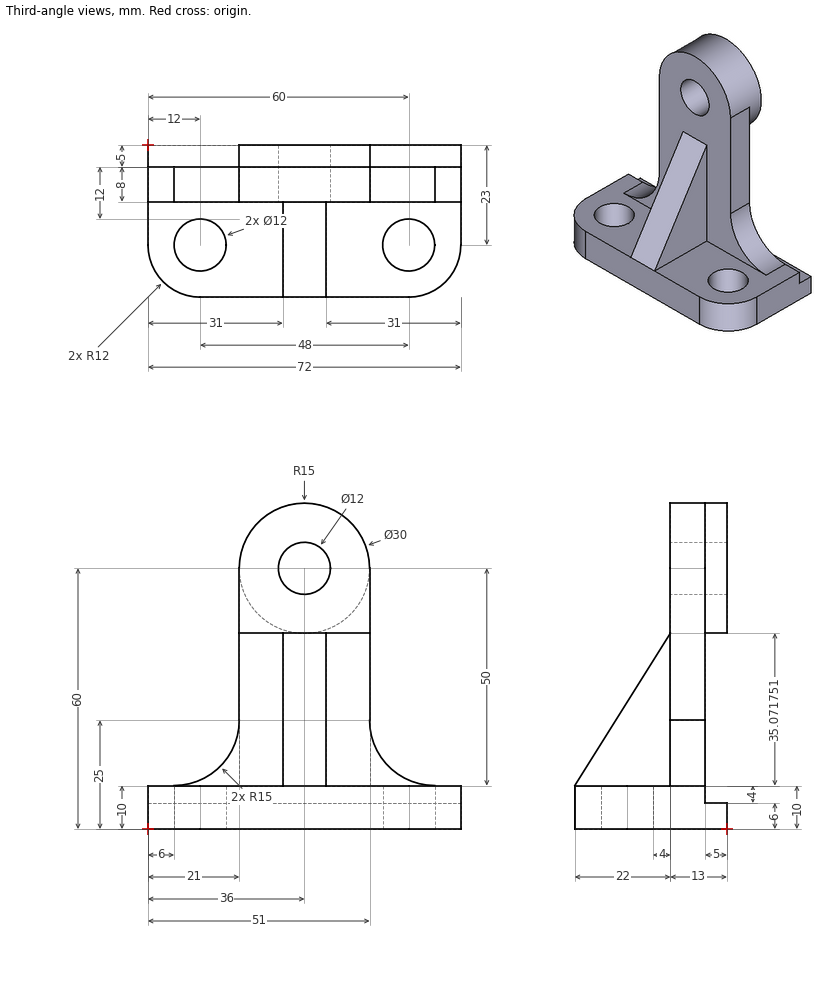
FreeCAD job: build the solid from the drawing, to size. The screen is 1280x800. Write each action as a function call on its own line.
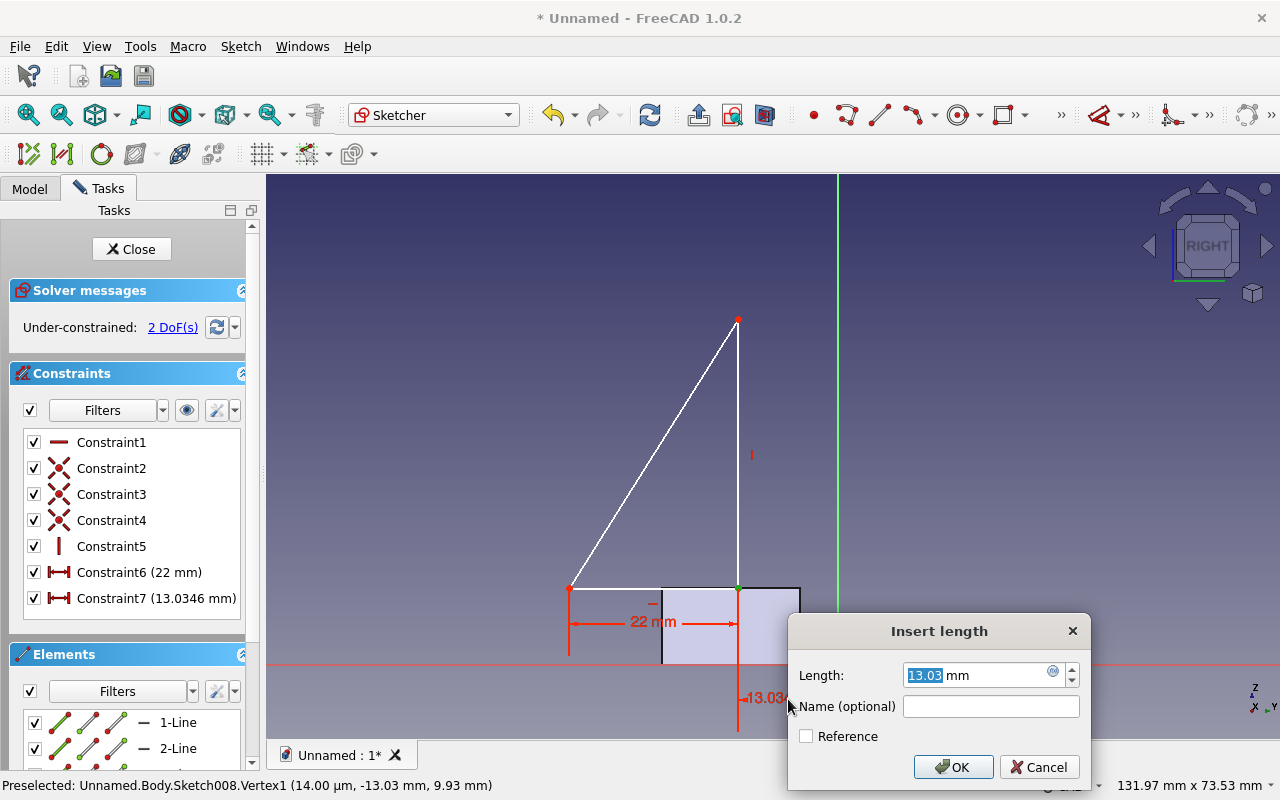
text(13)
key(Return)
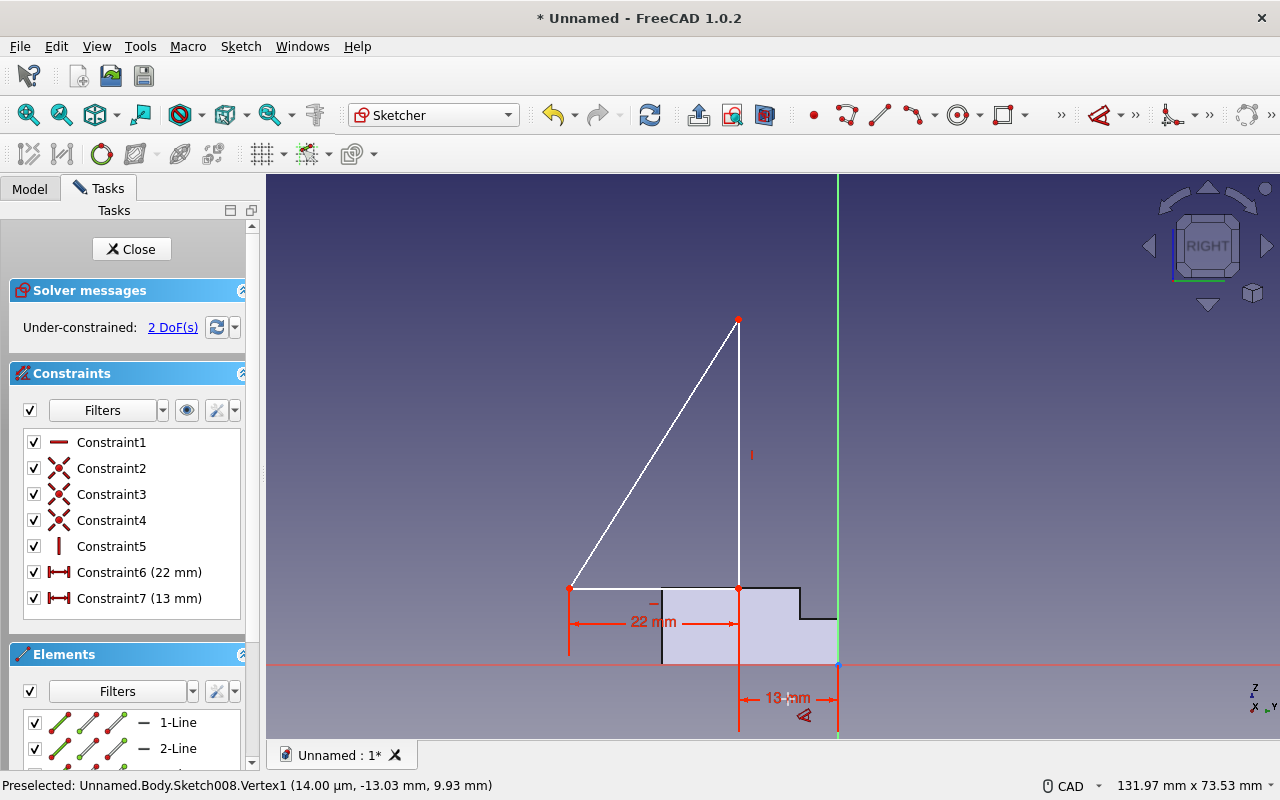
click(739, 589)
click(872, 627)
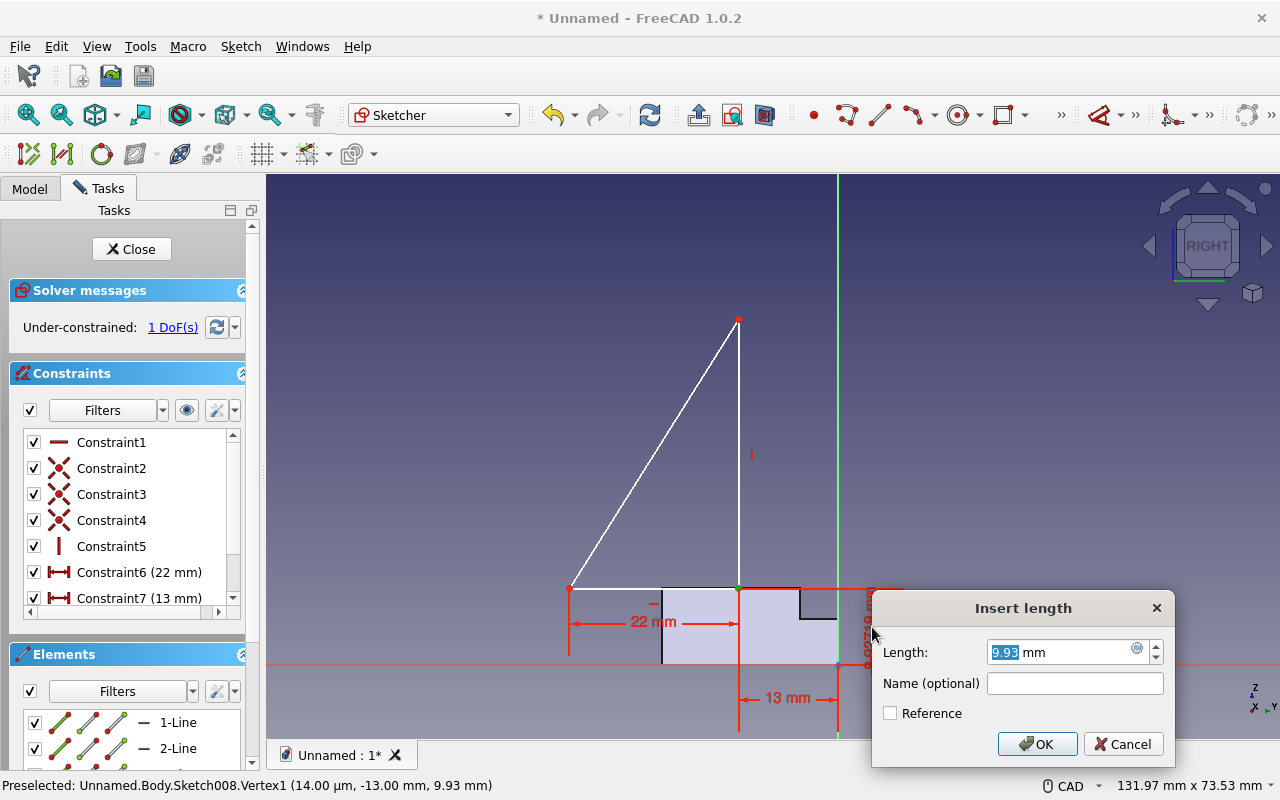
text(10)
key(Return)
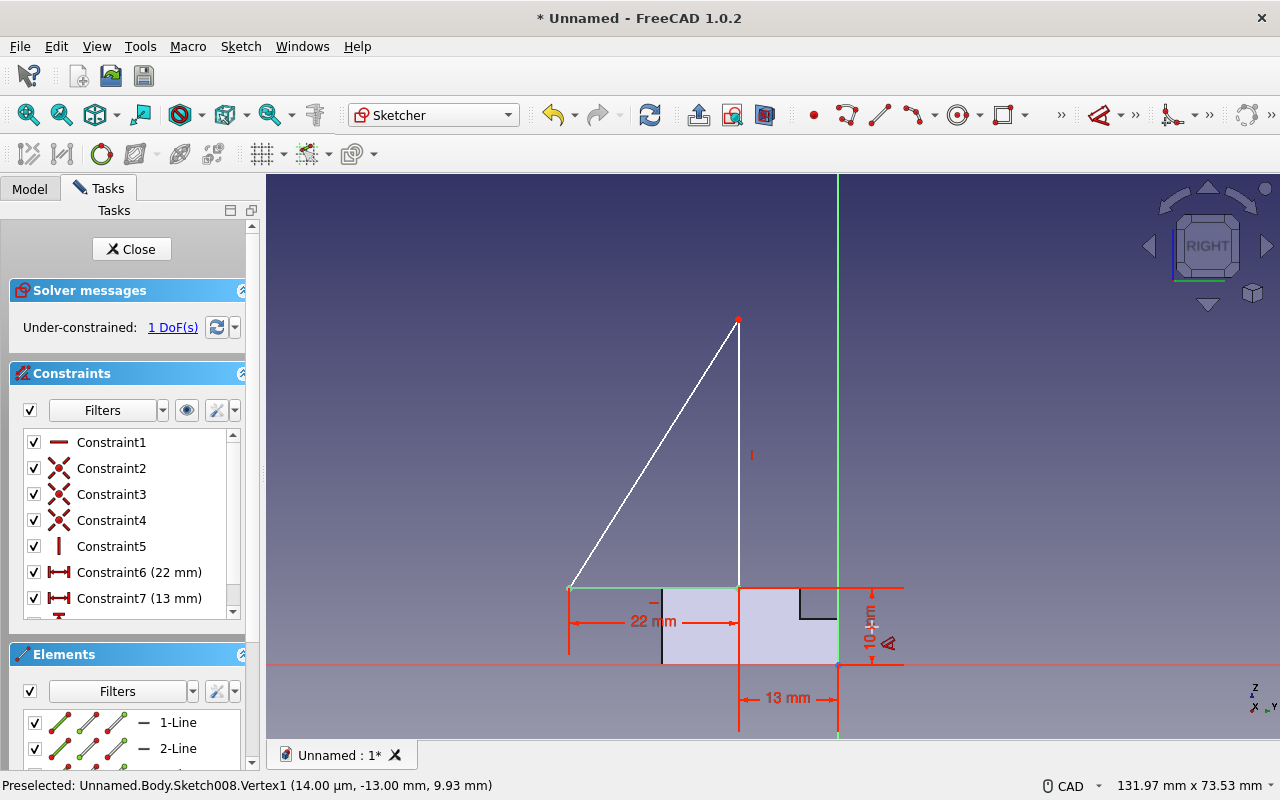
click(739, 401)
click(773, 454)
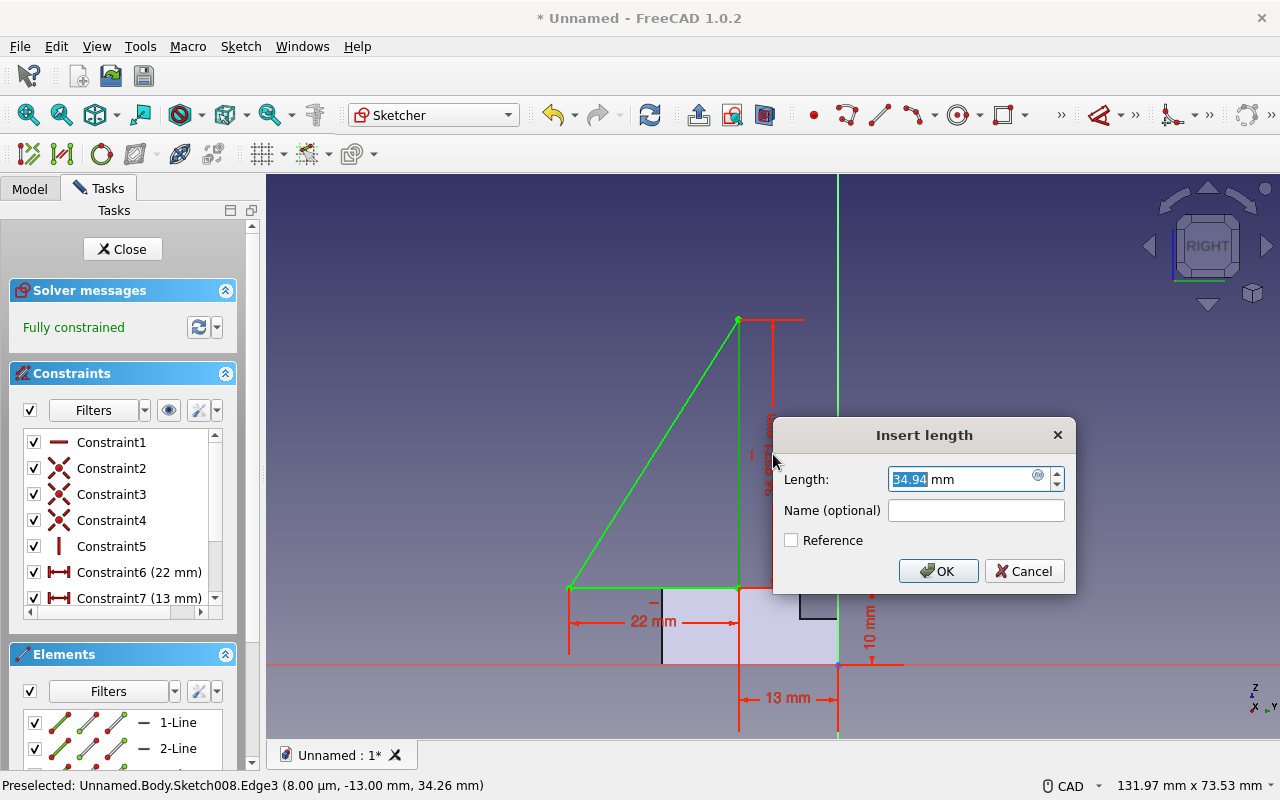
text(35.071751)
key(Return)
key(Escape)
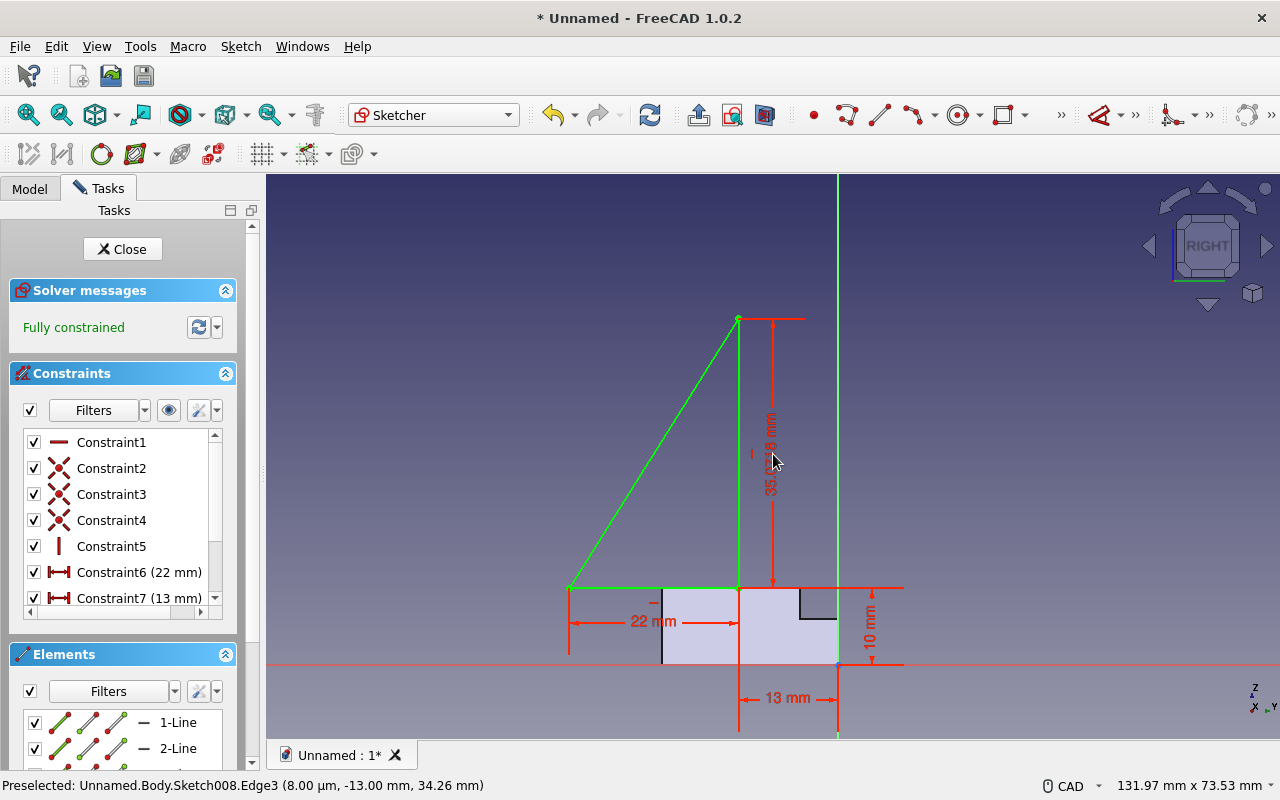
click(123, 249)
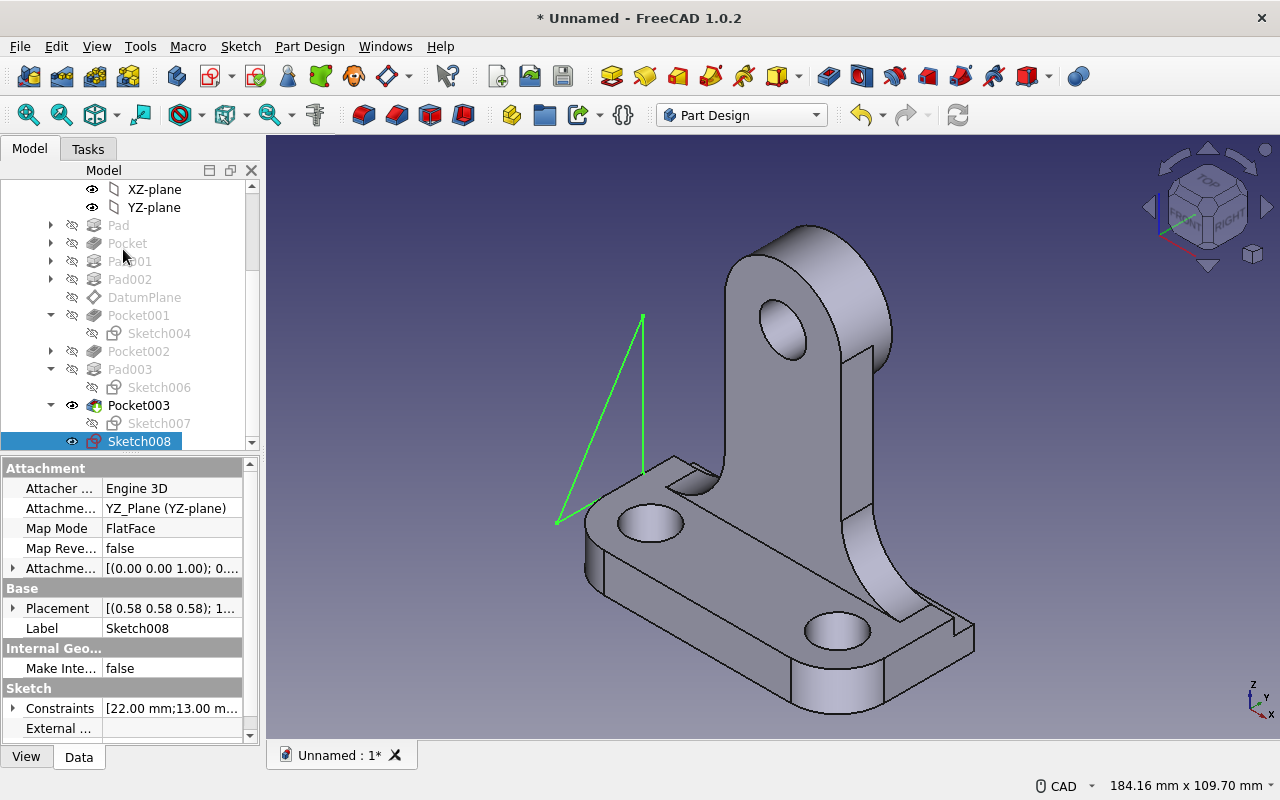
click(612, 76)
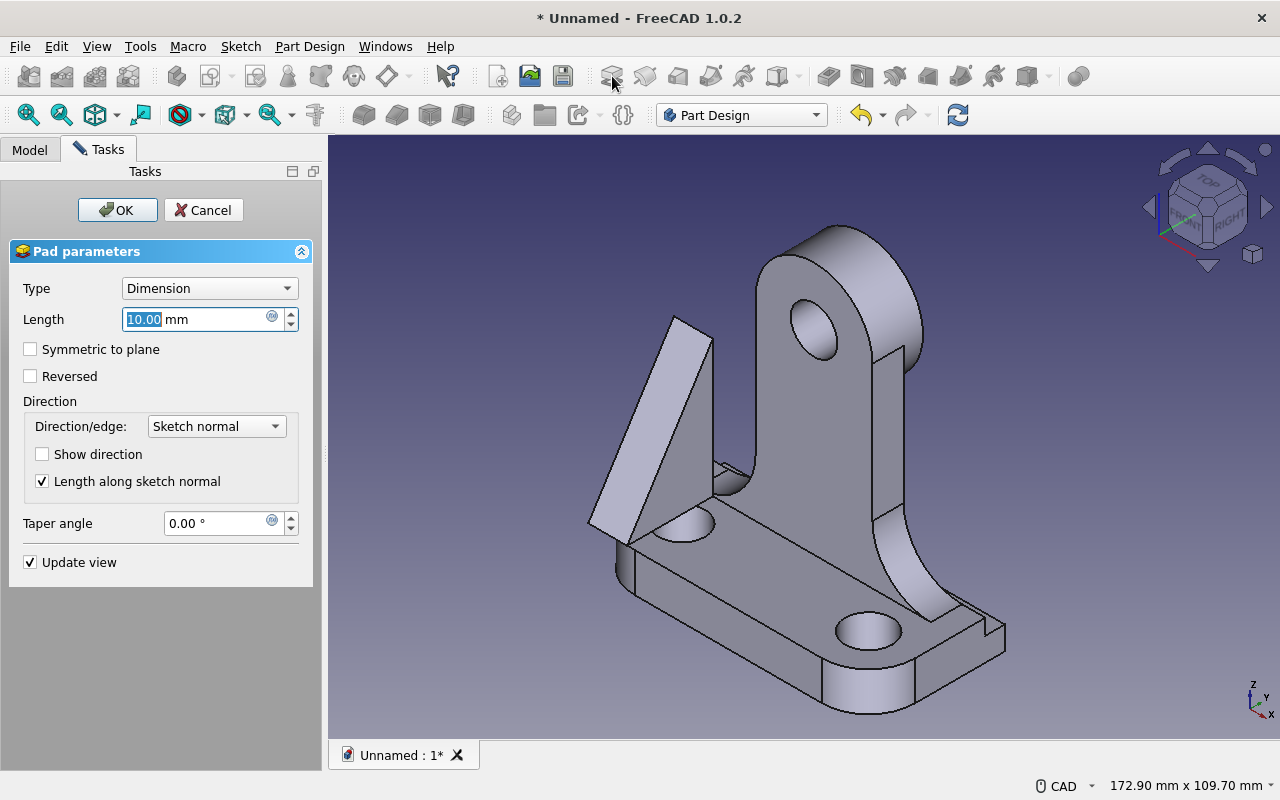
text(72)
key(Tab)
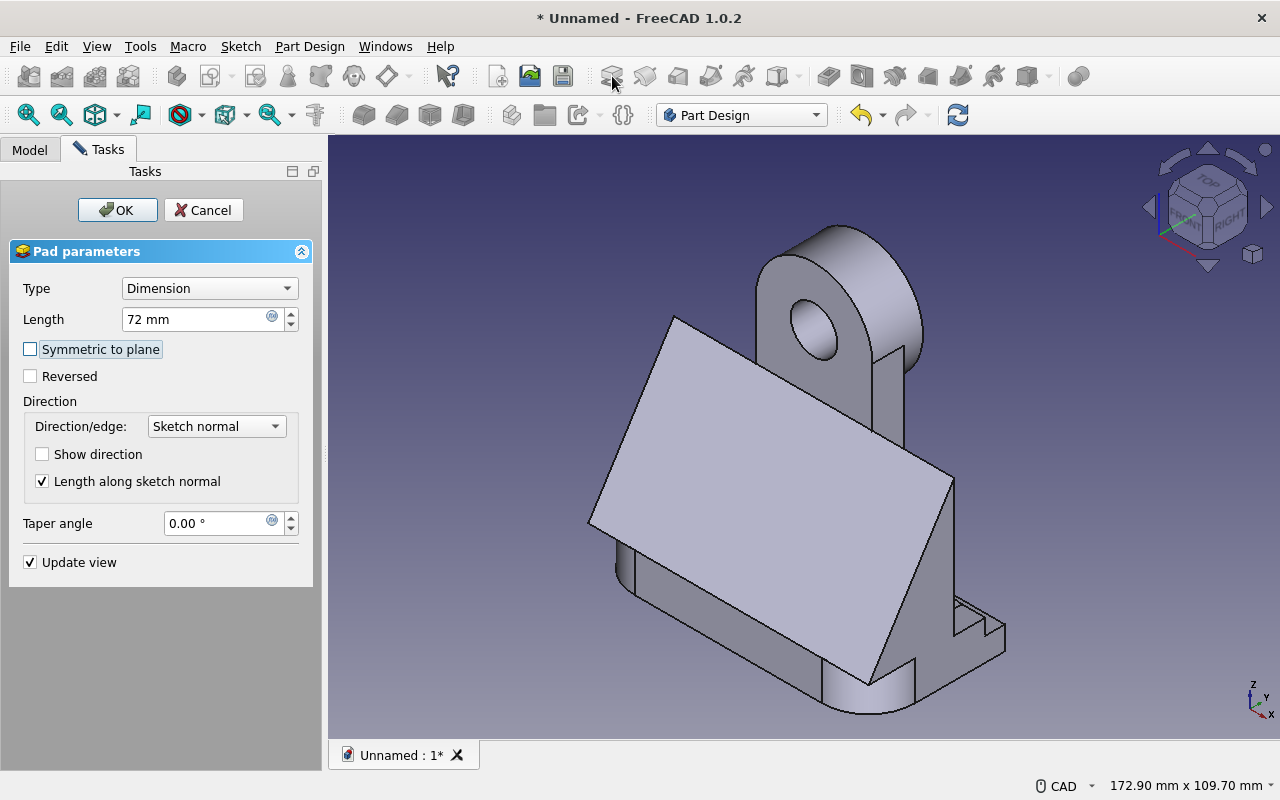
click(118, 210)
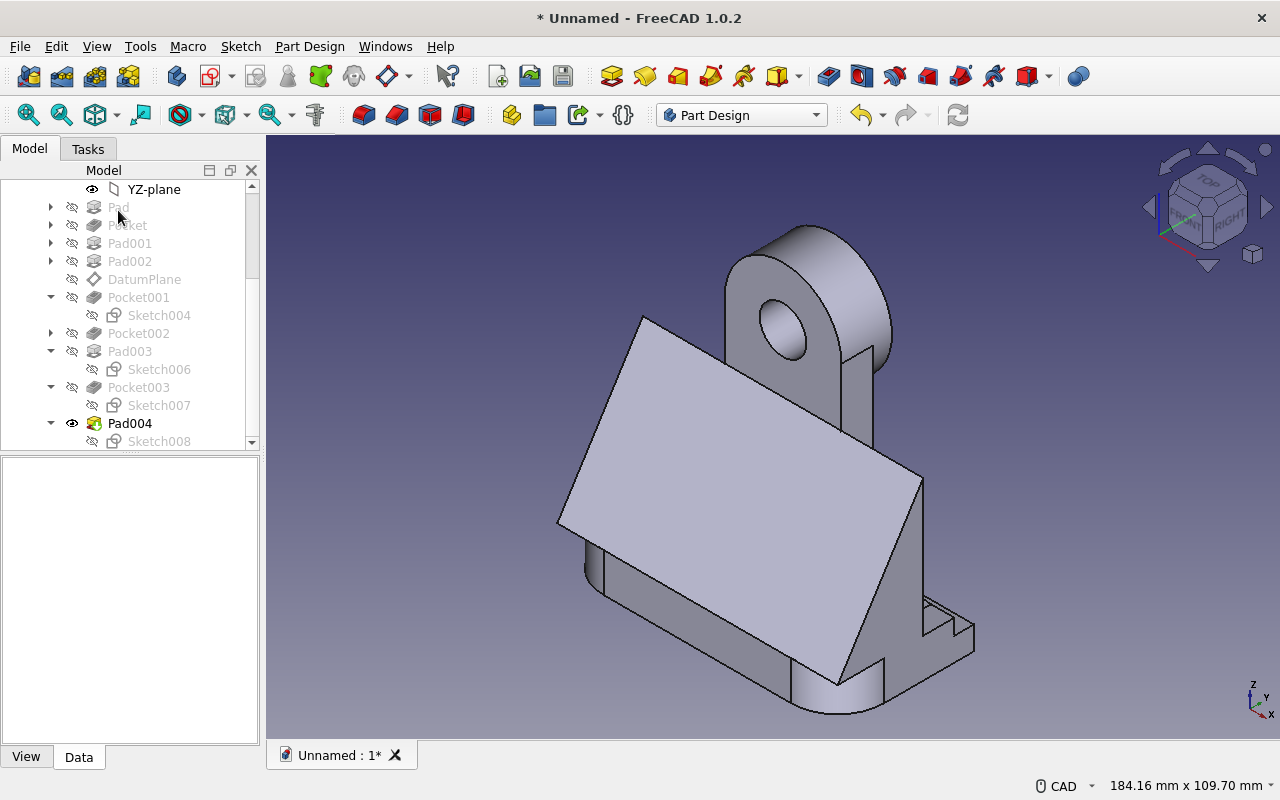
click(886, 629)